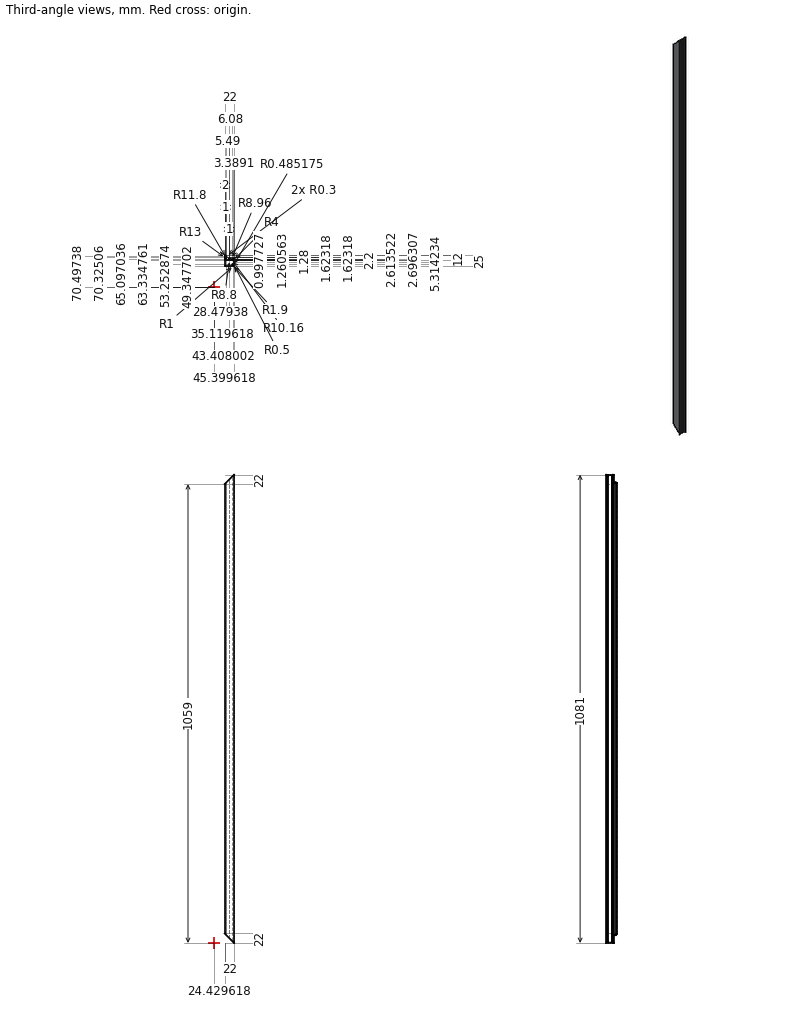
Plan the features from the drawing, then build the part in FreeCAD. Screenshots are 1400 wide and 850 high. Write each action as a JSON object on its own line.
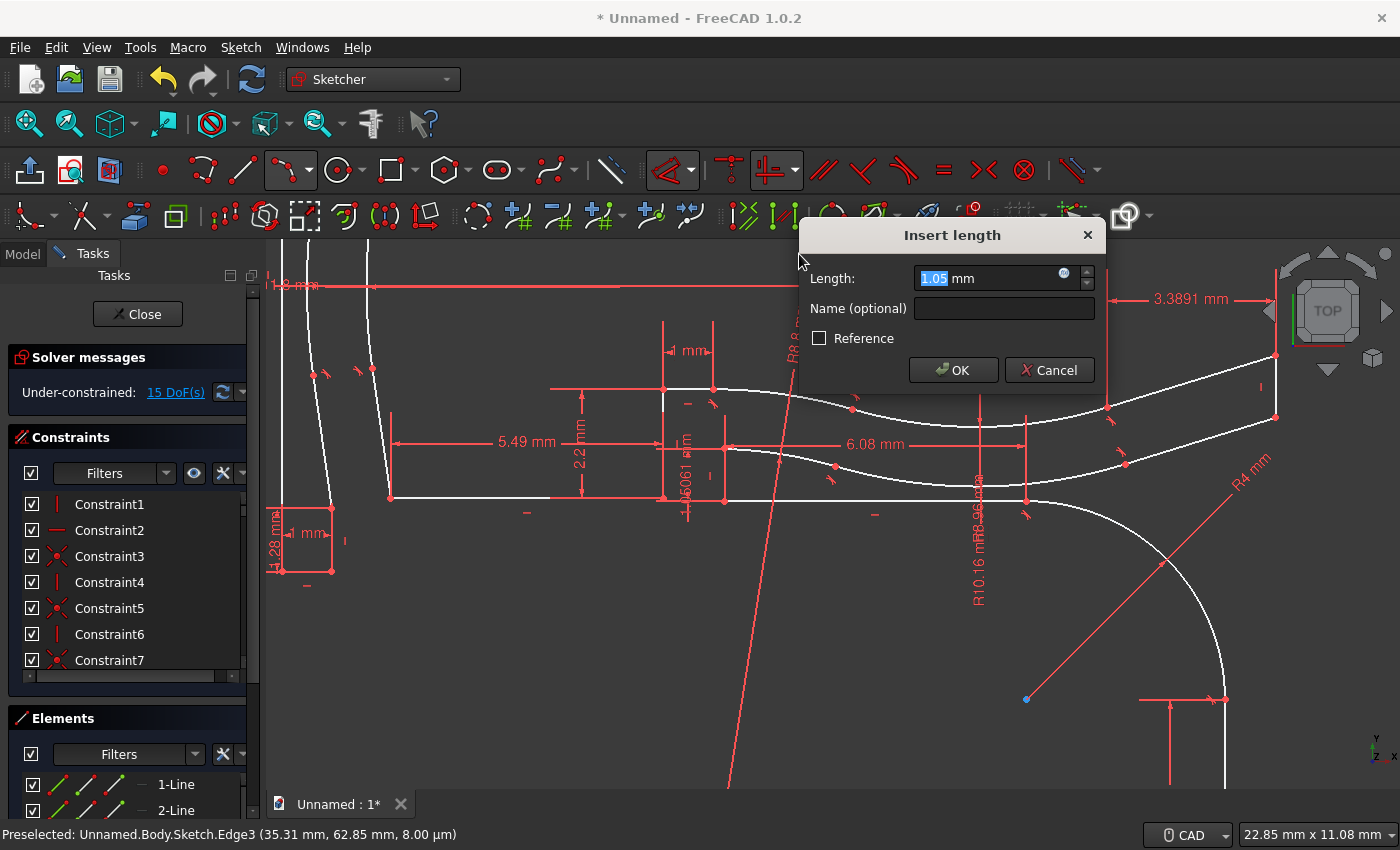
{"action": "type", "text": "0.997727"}
{"action": "key", "text": "Return"}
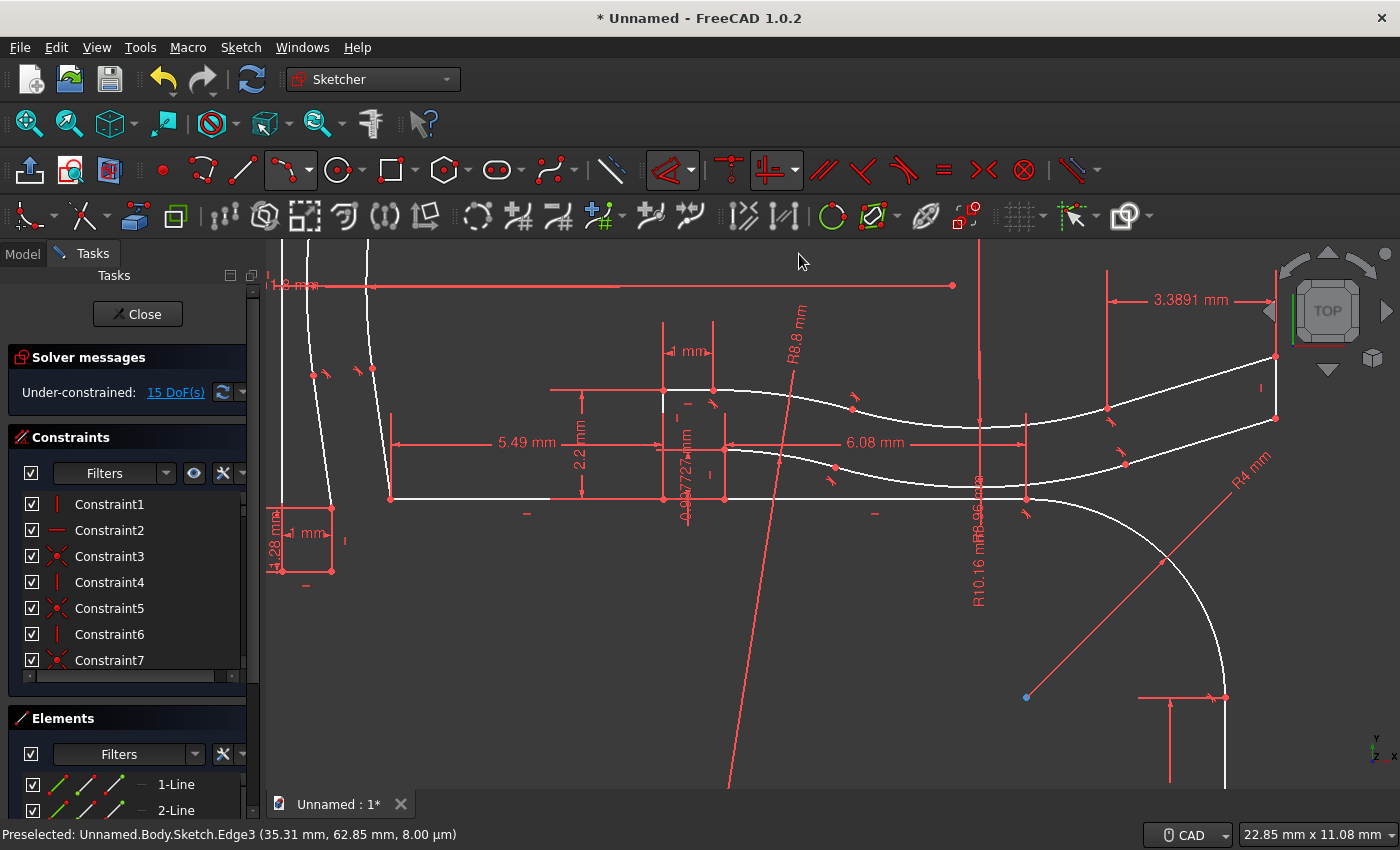
{"action": "scroll", "coordinate": [779, 480], "scroll_direction": "down", "scroll_amount": 6}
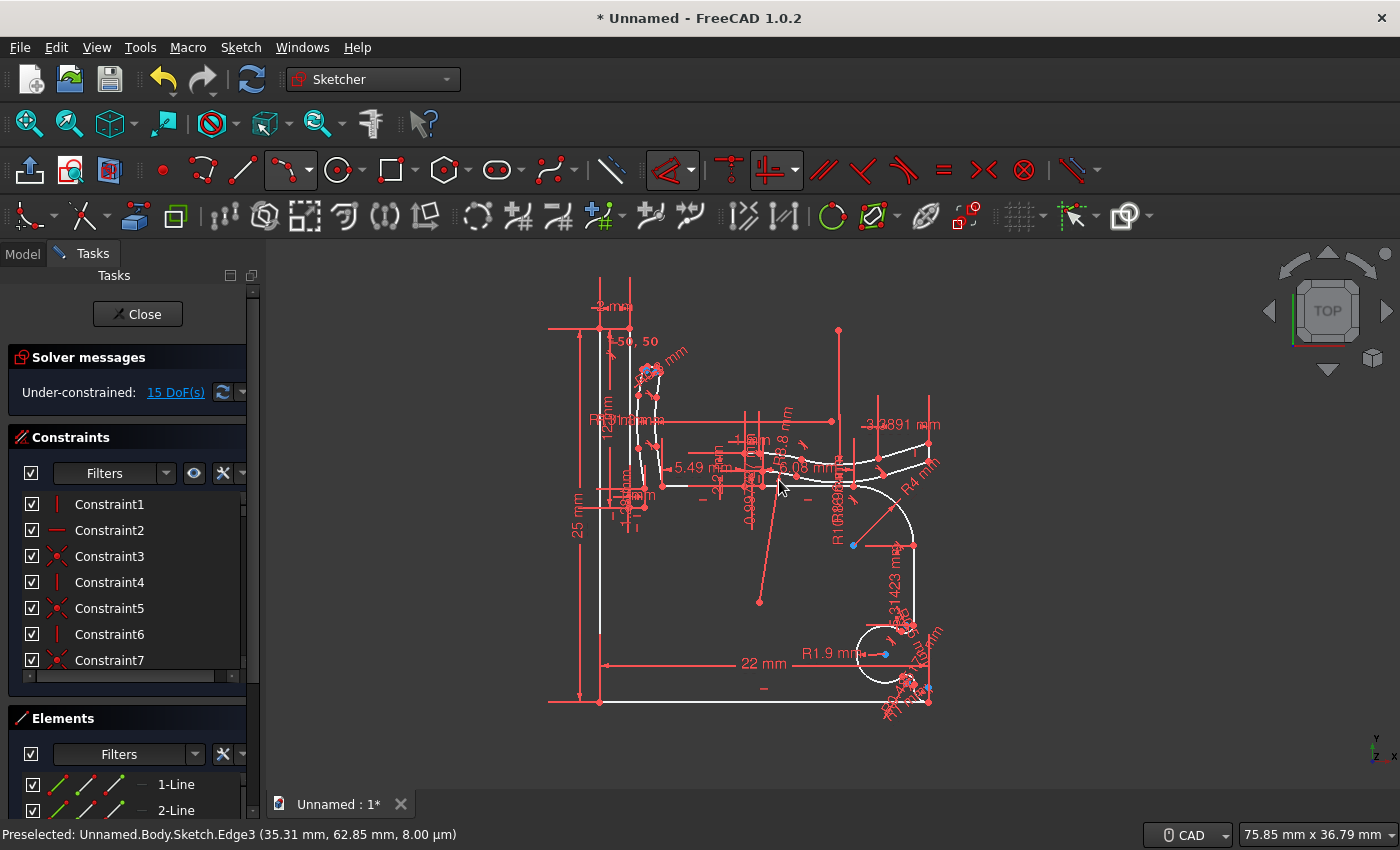
{"action": "scroll", "coordinate": [929, 456], "scroll_direction": "up", "scroll_amount": 5}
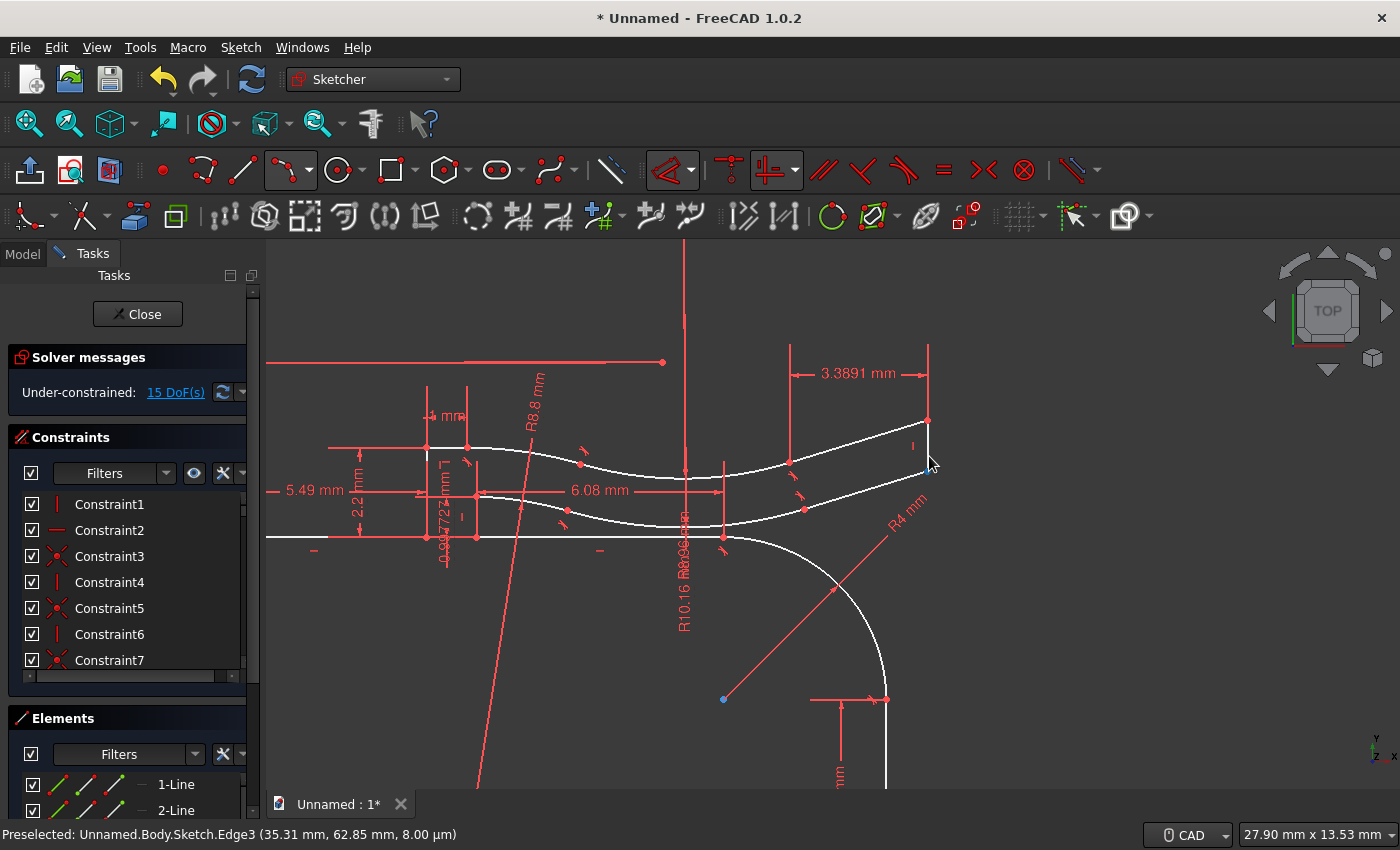
{"action": "left_click", "coordinate": [928, 456]}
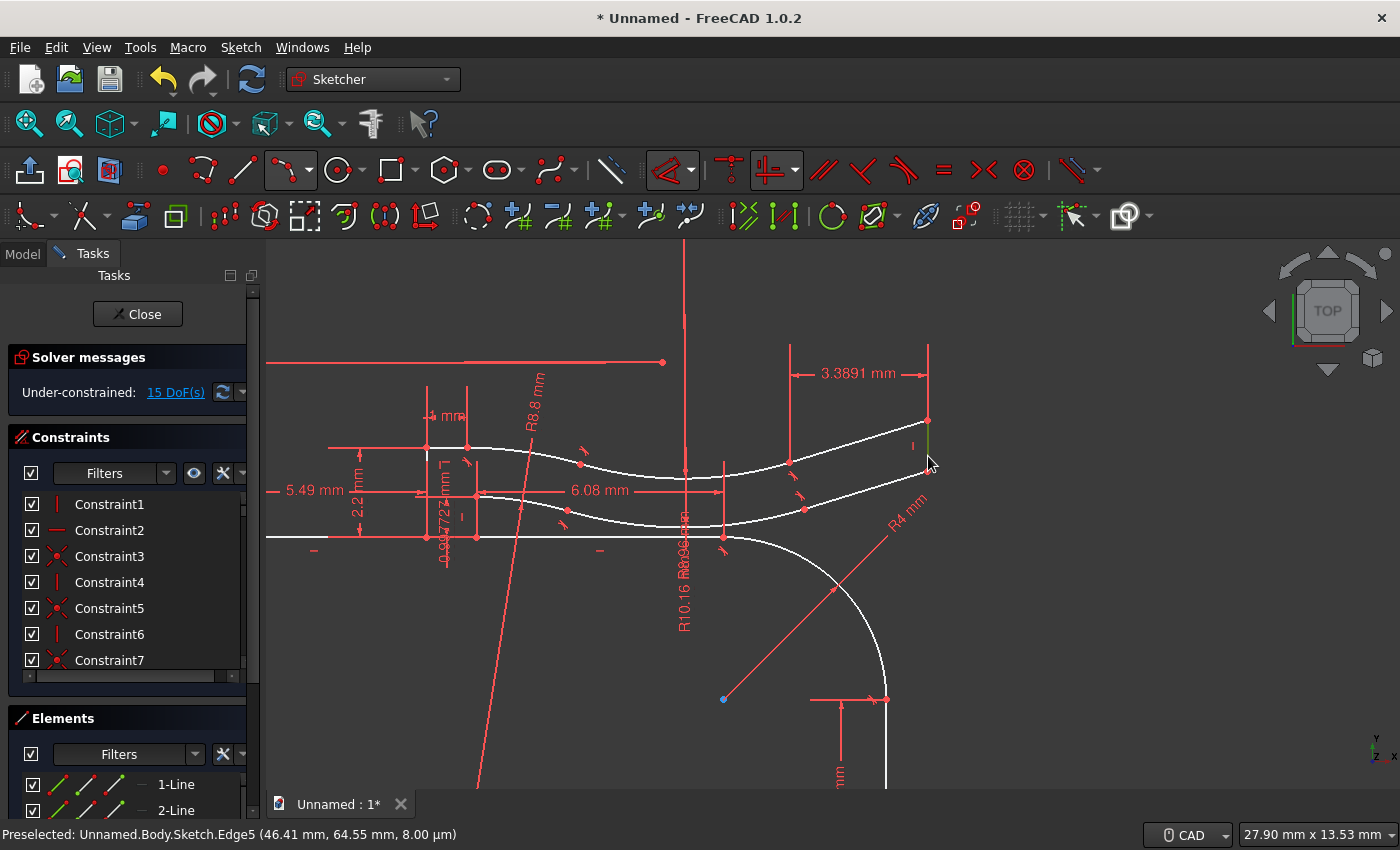
{"action": "key", "text": "i"}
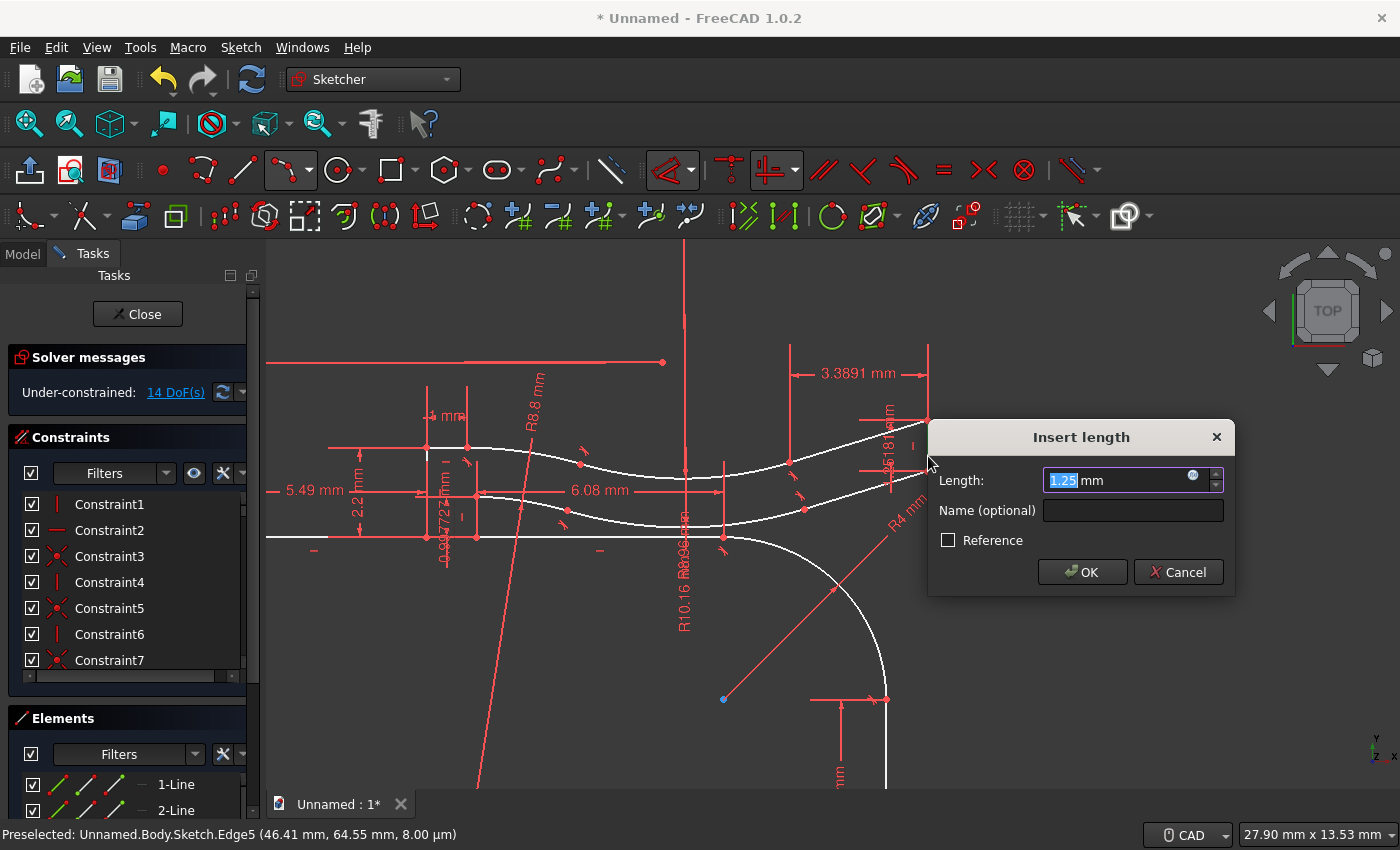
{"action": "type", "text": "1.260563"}
{"action": "key", "text": "Return"}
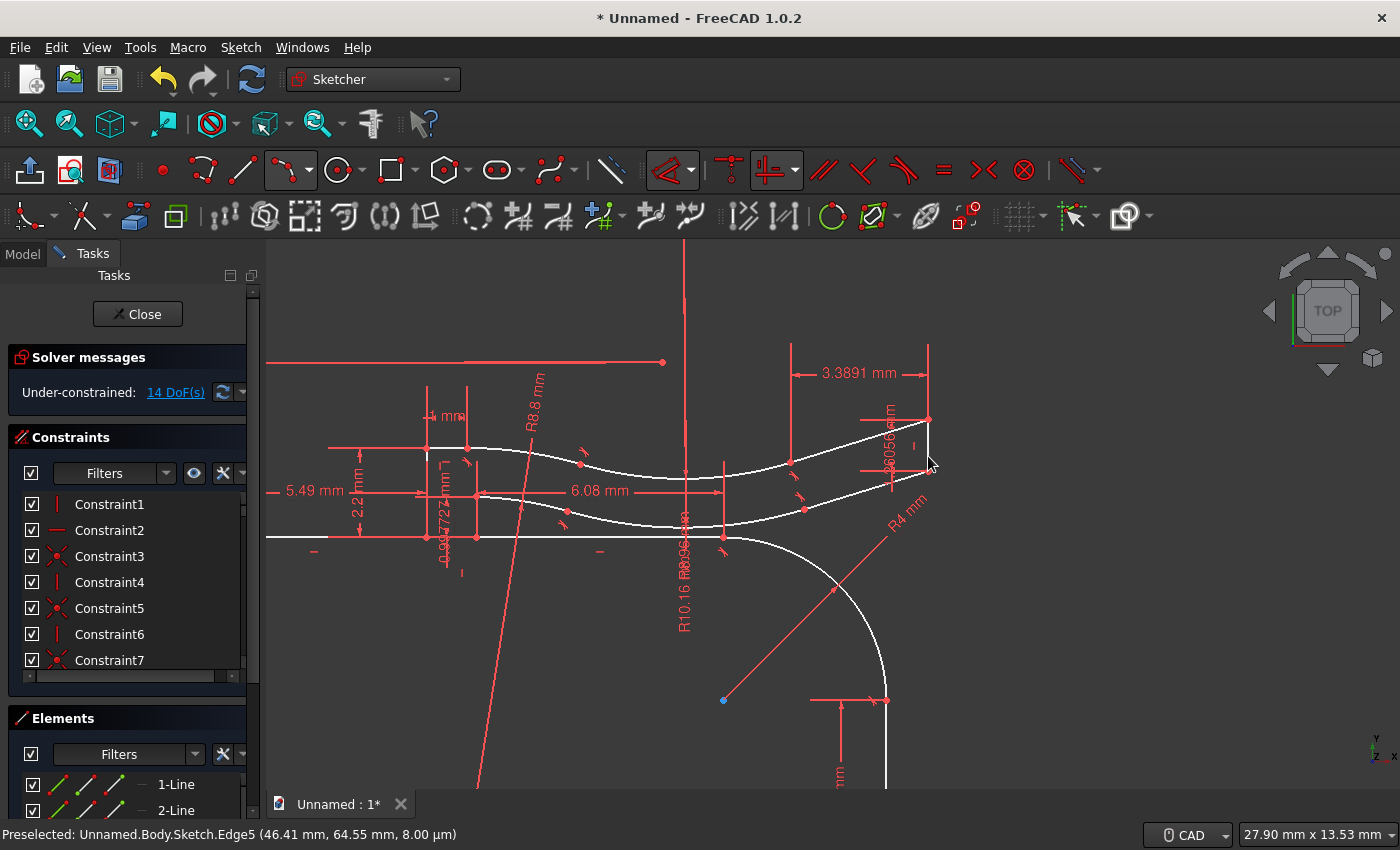
{"action": "scroll", "coordinate": [929, 456], "scroll_direction": "down", "scroll_amount": 5}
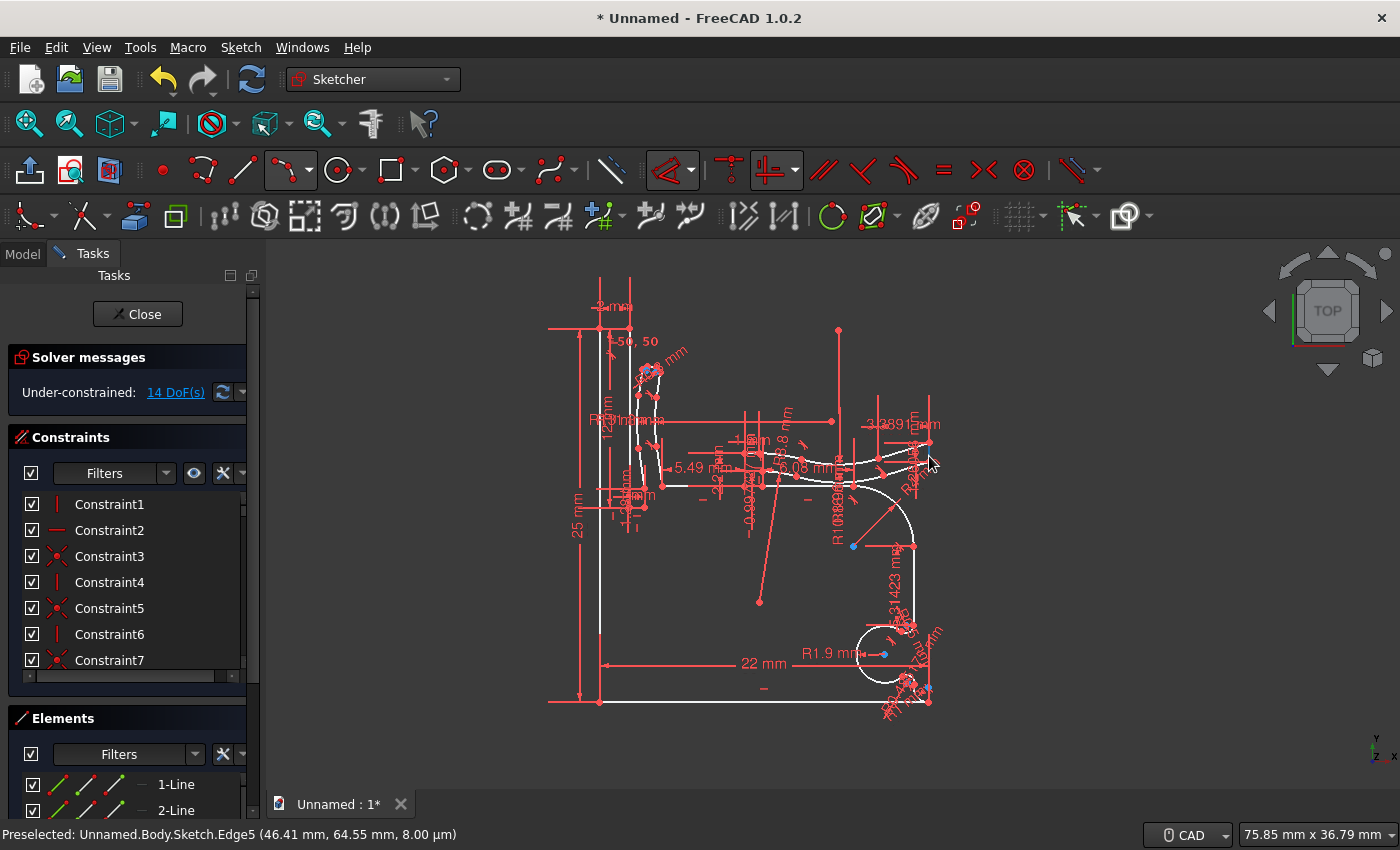
{"action": "scroll", "coordinate": [658, 390], "scroll_direction": "up", "scroll_amount": 4}